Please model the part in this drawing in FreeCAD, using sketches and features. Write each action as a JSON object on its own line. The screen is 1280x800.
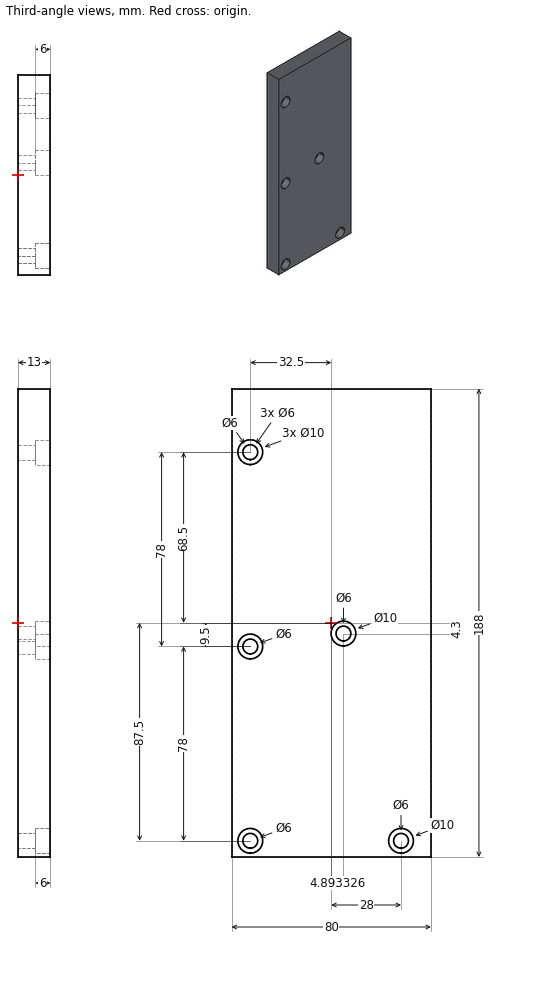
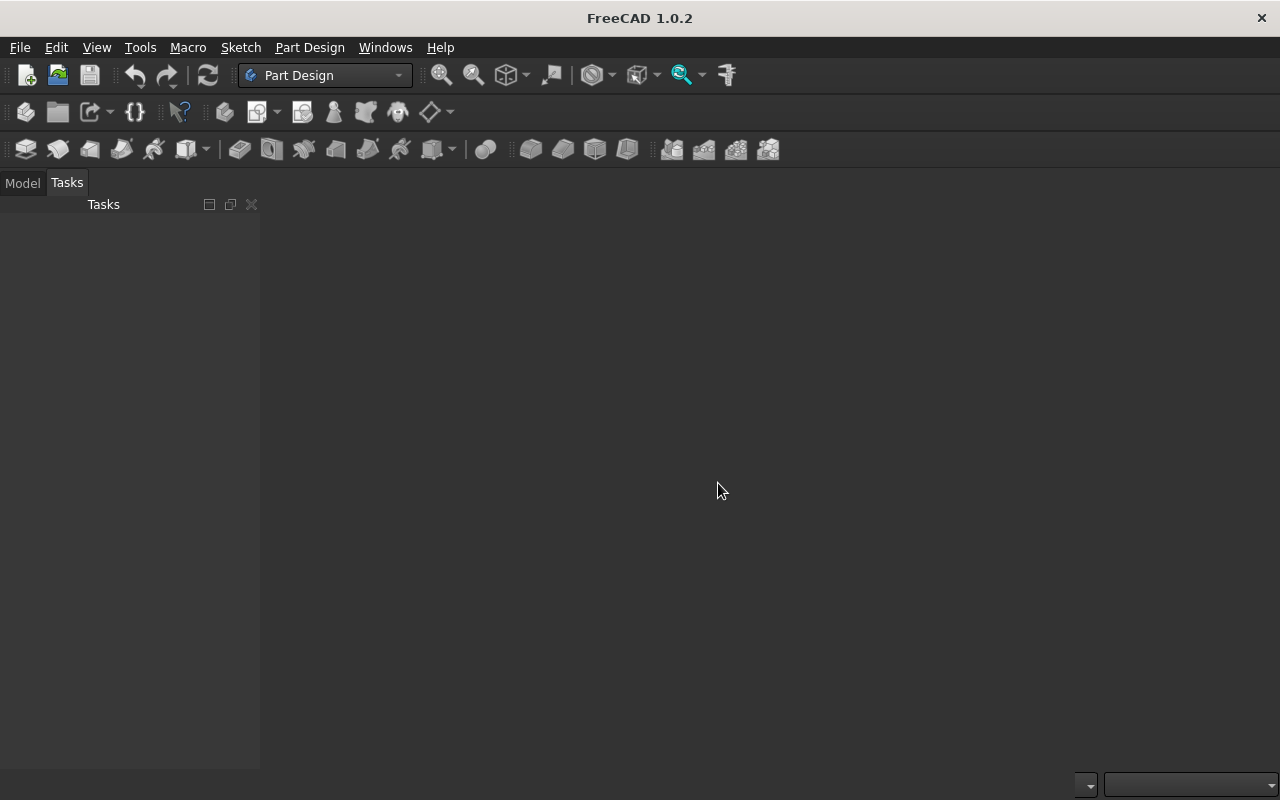
{"action": "left_click", "coordinate": [26, 76]}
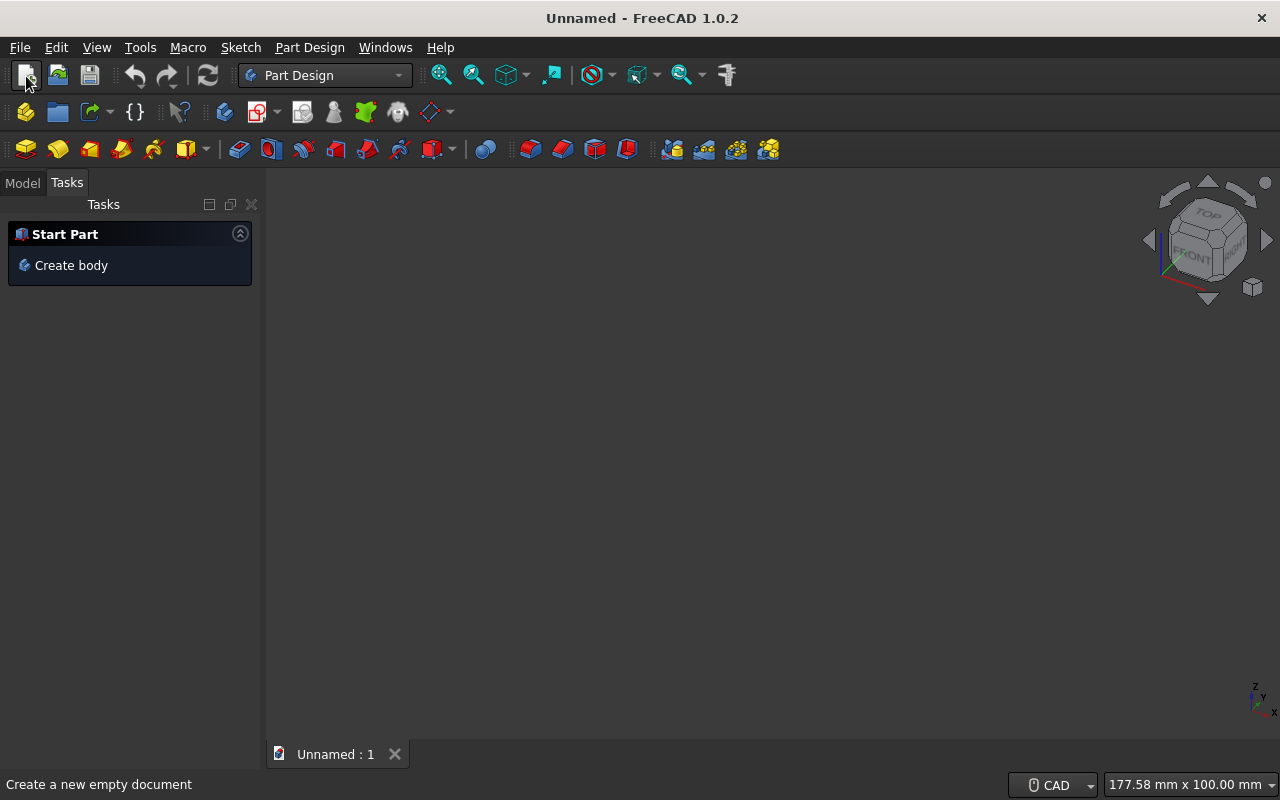
{"action": "left_click", "coordinate": [258, 112]}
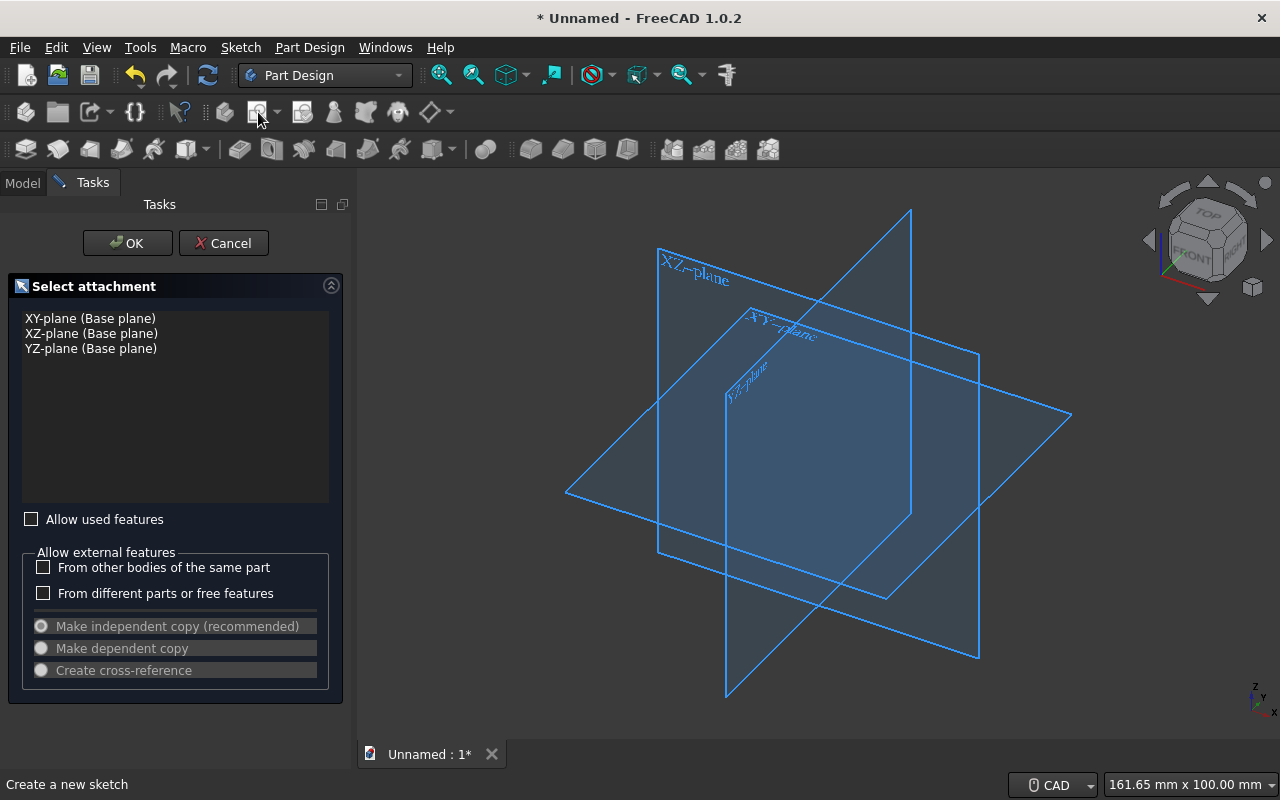
{"action": "left_click", "coordinate": [82, 348]}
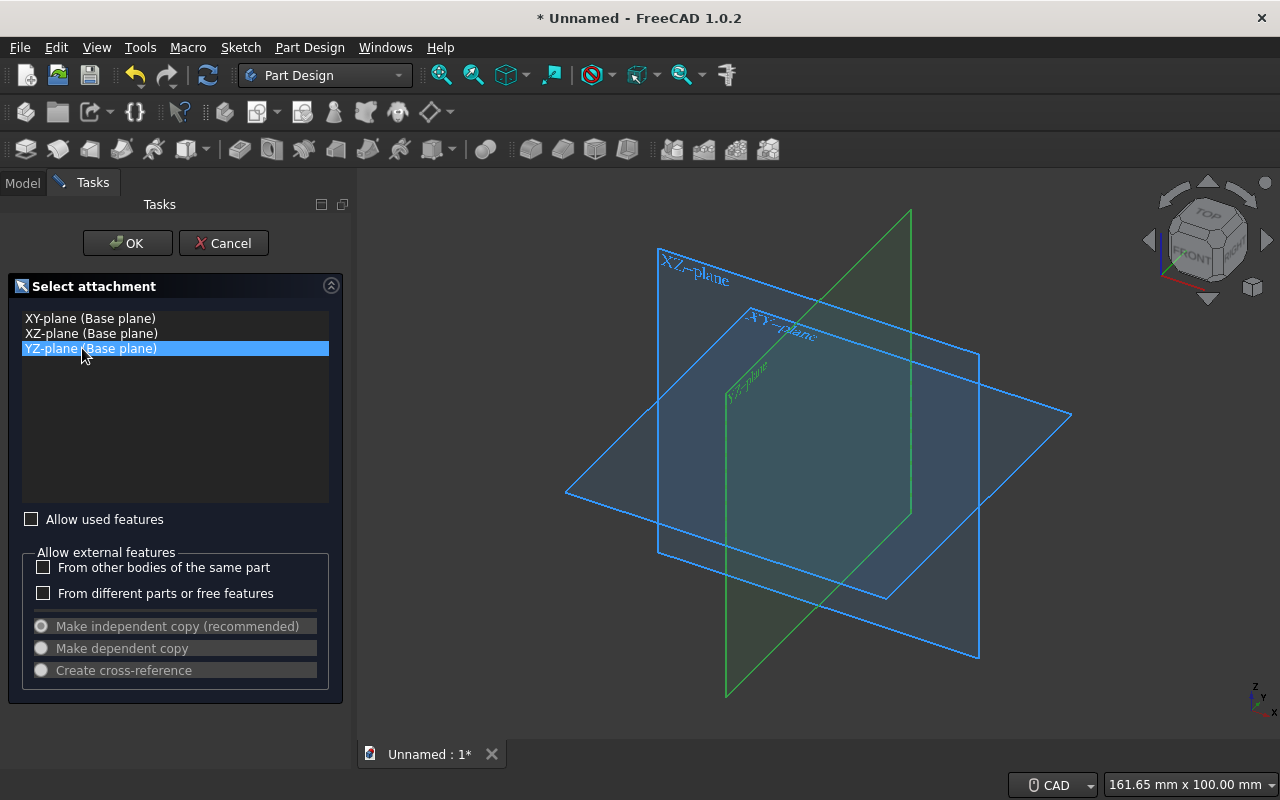
{"action": "left_click", "coordinate": [128, 243]}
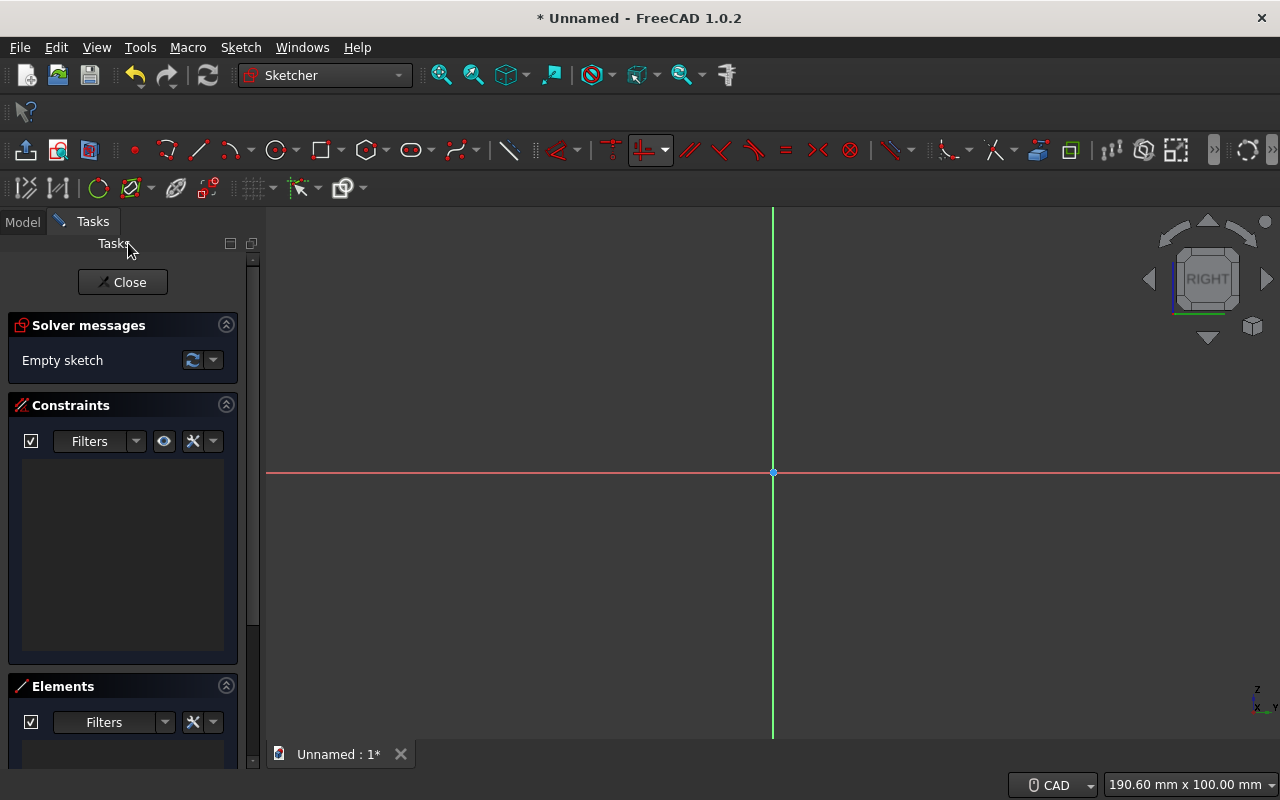
{"action": "scroll", "coordinate": [665, 473], "scroll_direction": "down", "scroll_amount": 5}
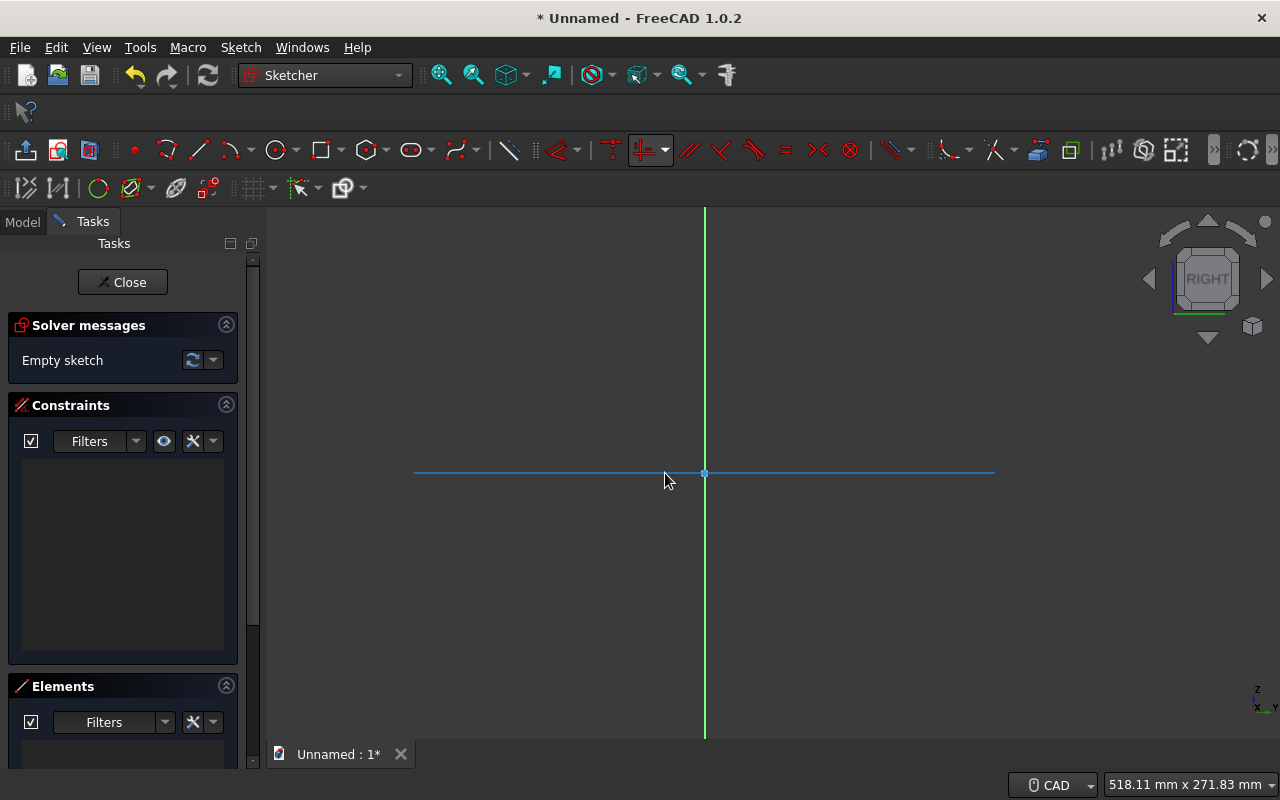
{"action": "key", "text": "g v"}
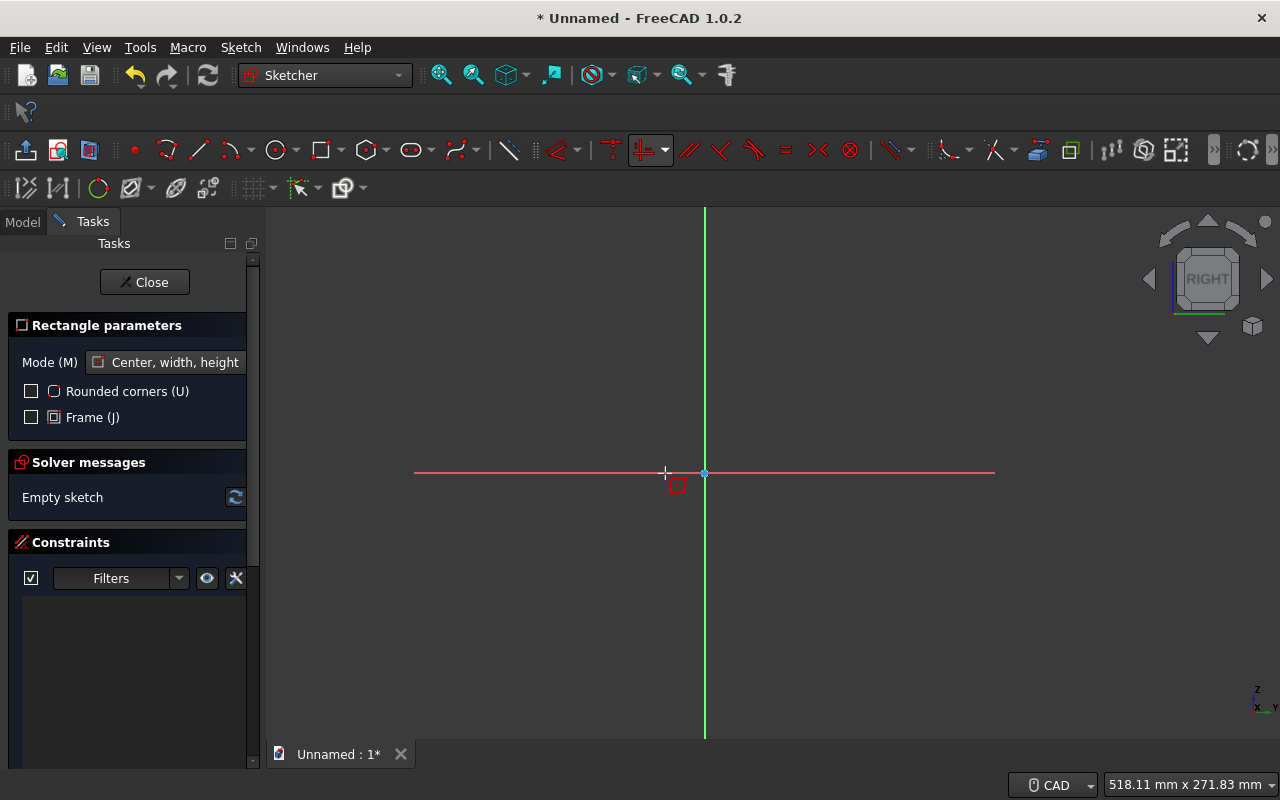
{"action": "left_click", "coordinate": [705, 473]}
{"action": "left_click", "coordinate": [783, 289]}
{"action": "key", "text": "Escape"}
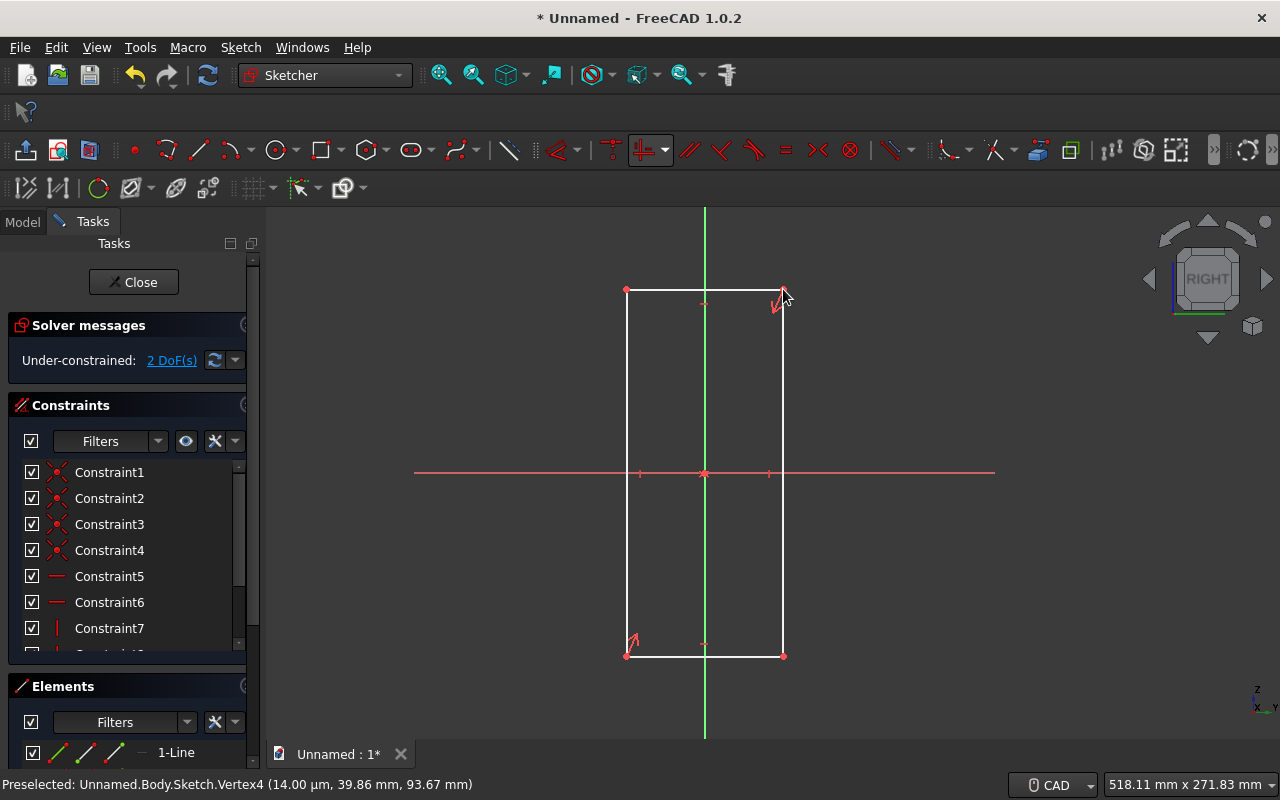
{"action": "left_click", "coordinate": [674, 657]}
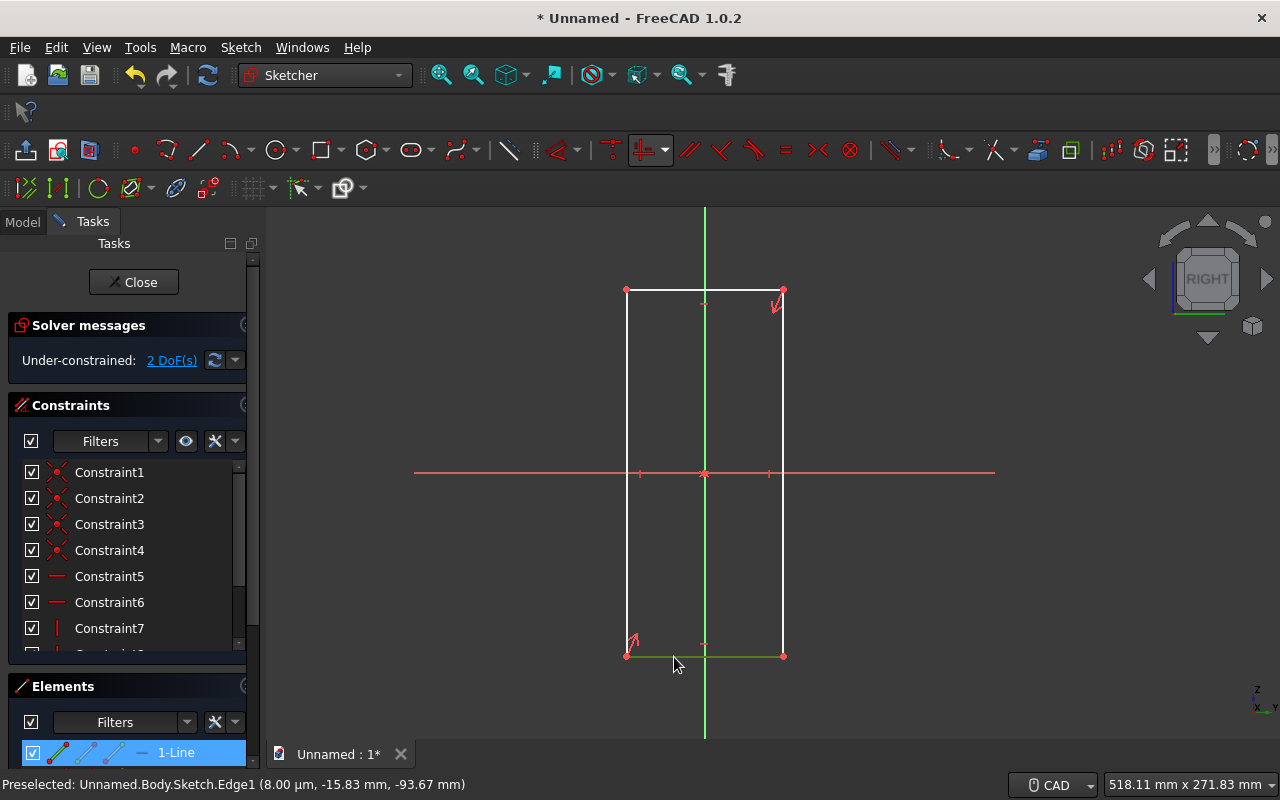
{"action": "key", "text": "l"}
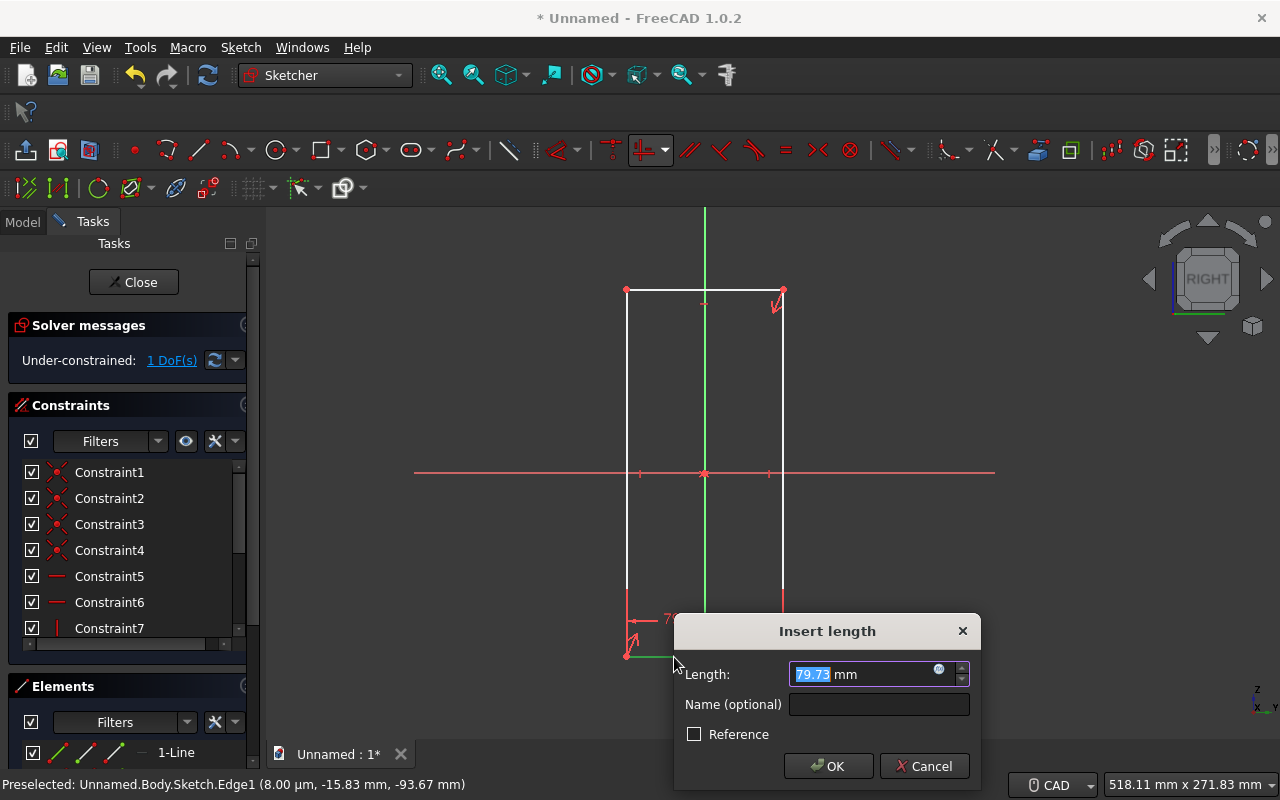
{"action": "type", "text": "80"}
{"action": "key", "text": "Return"}